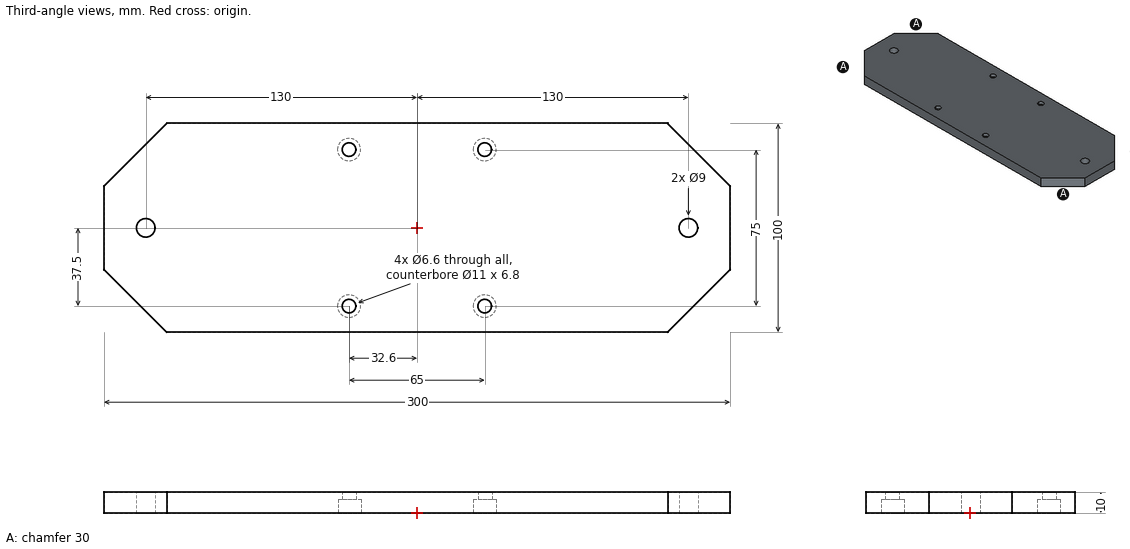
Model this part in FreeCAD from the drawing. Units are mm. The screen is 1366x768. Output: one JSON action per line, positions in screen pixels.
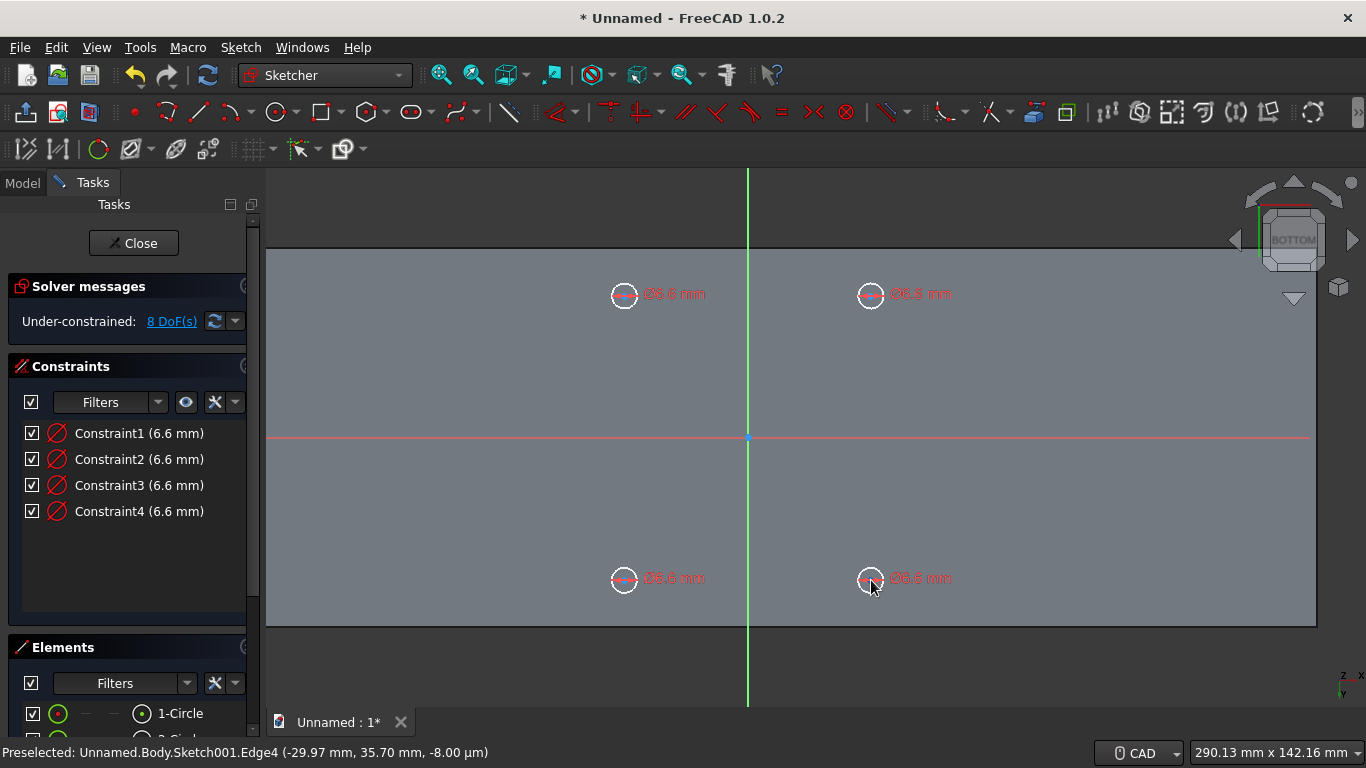
{"action": "left_click", "coordinate": [625, 296]}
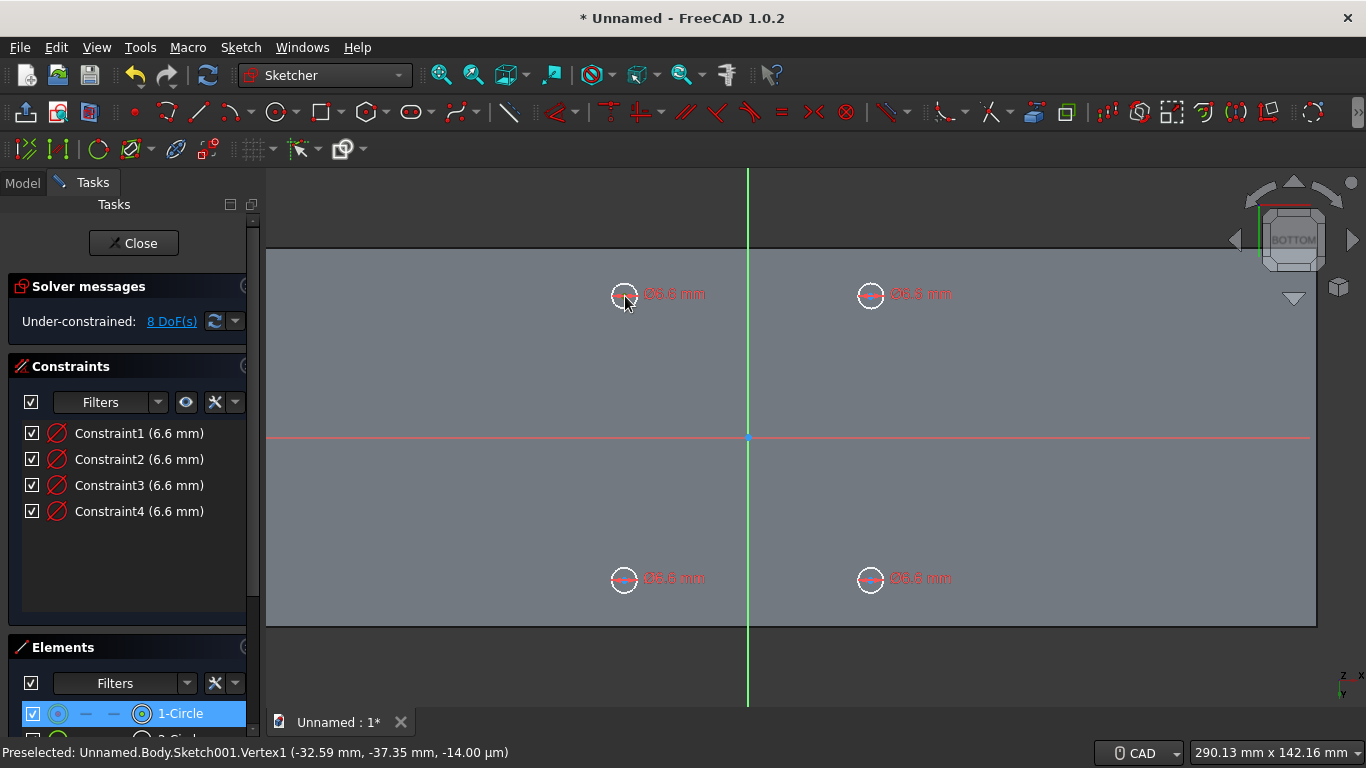
{"action": "left_click", "coordinate": [871, 296]}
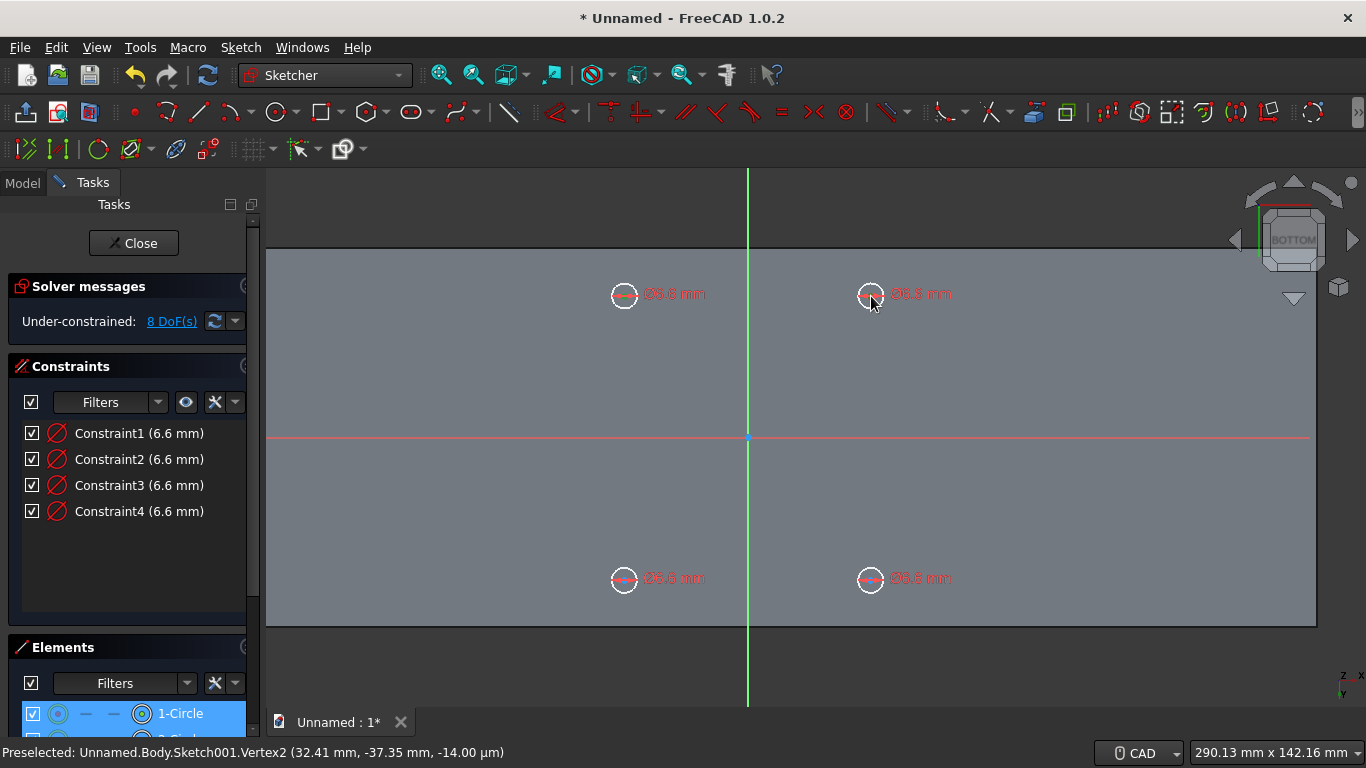
{"action": "key", "text": "h"}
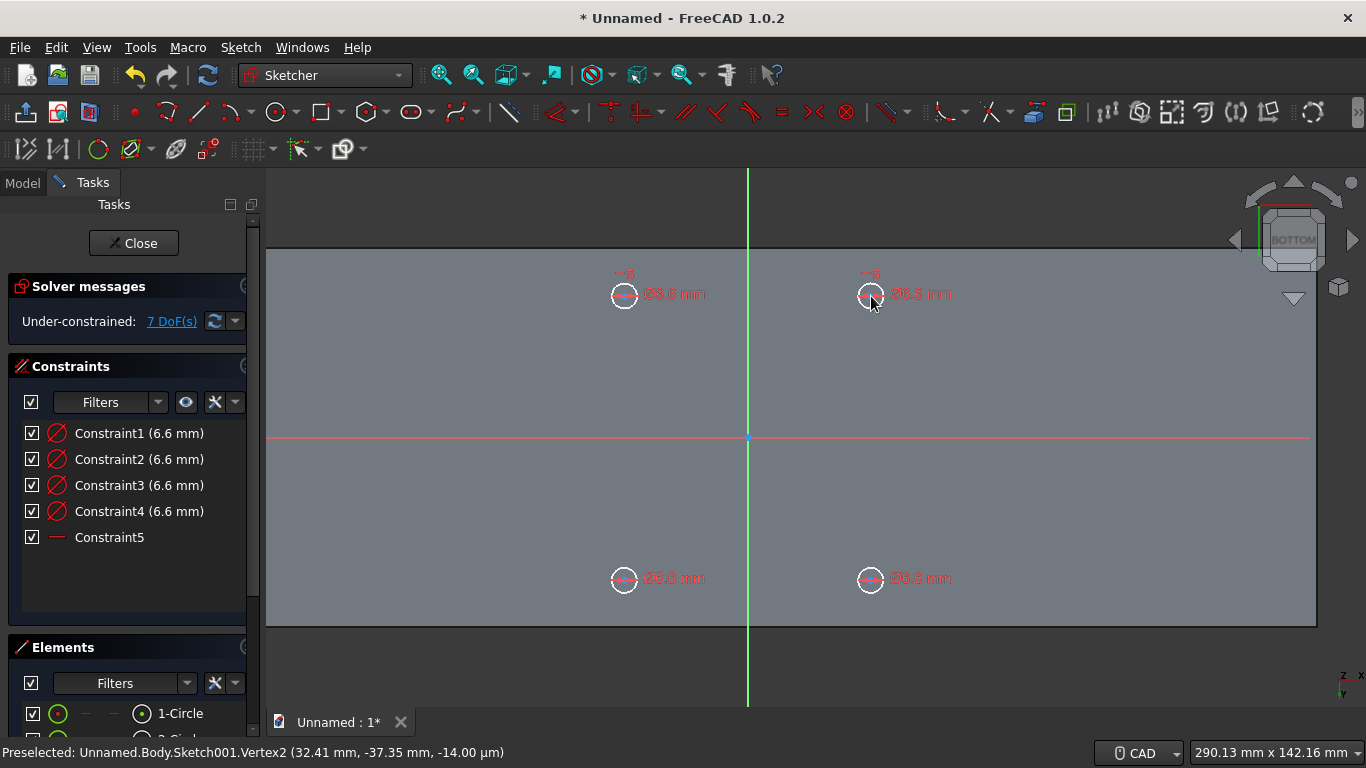
{"action": "left_click", "coordinate": [871, 296]}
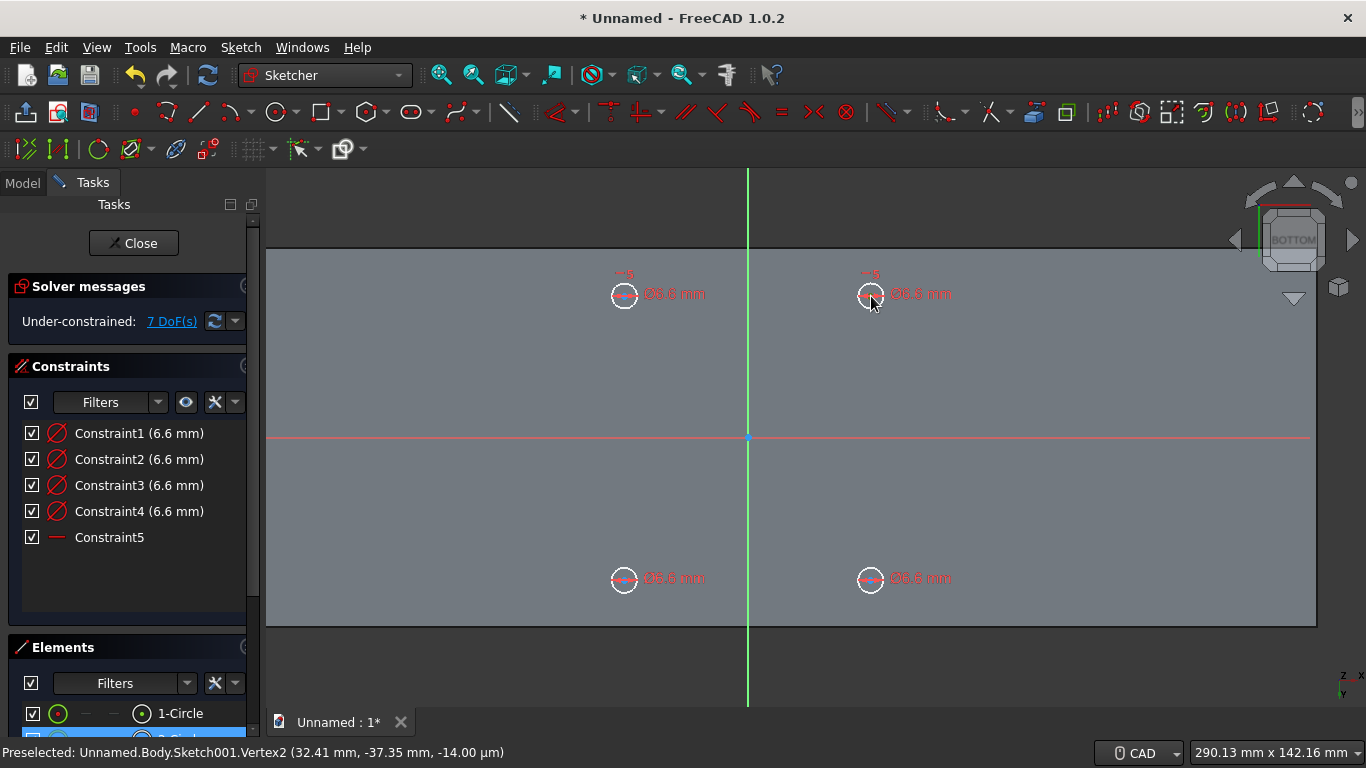
{"action": "left_click", "coordinate": [871, 580]}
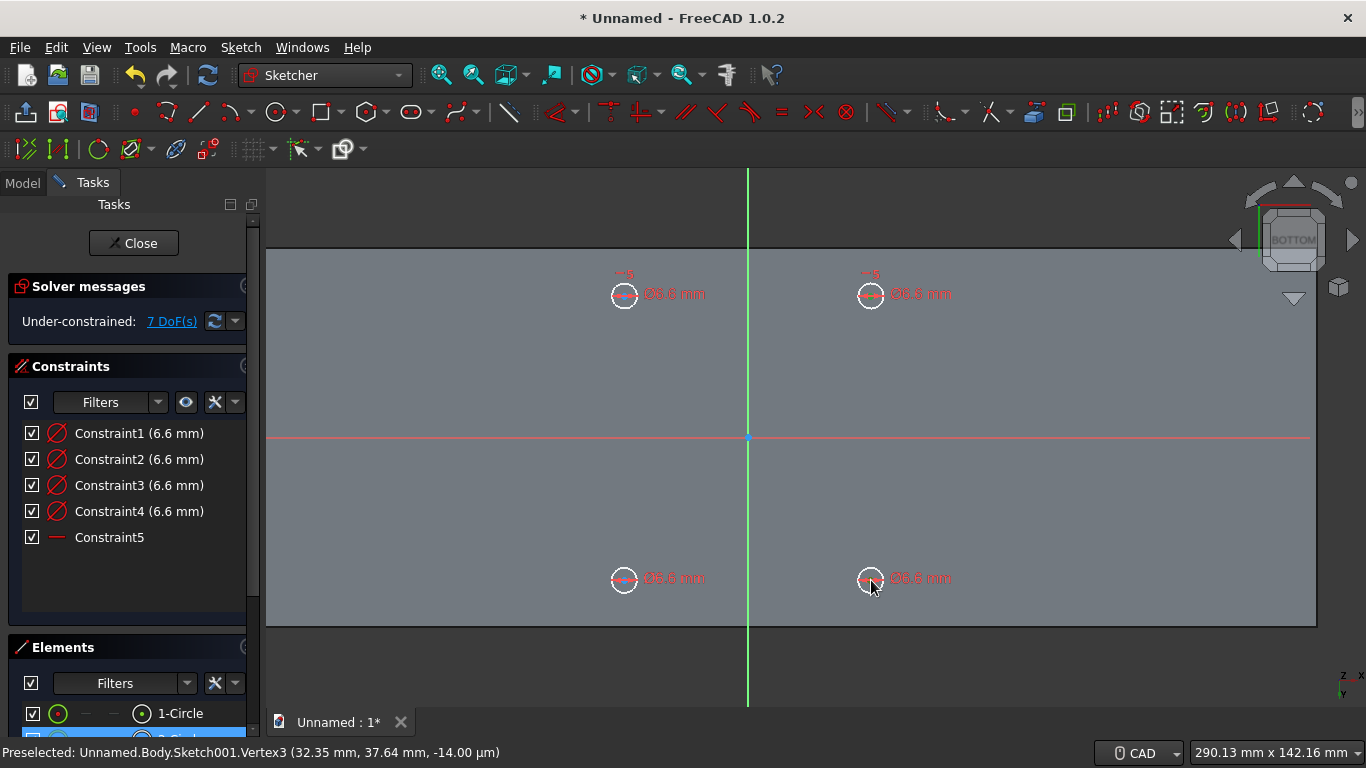
{"action": "key", "text": "v"}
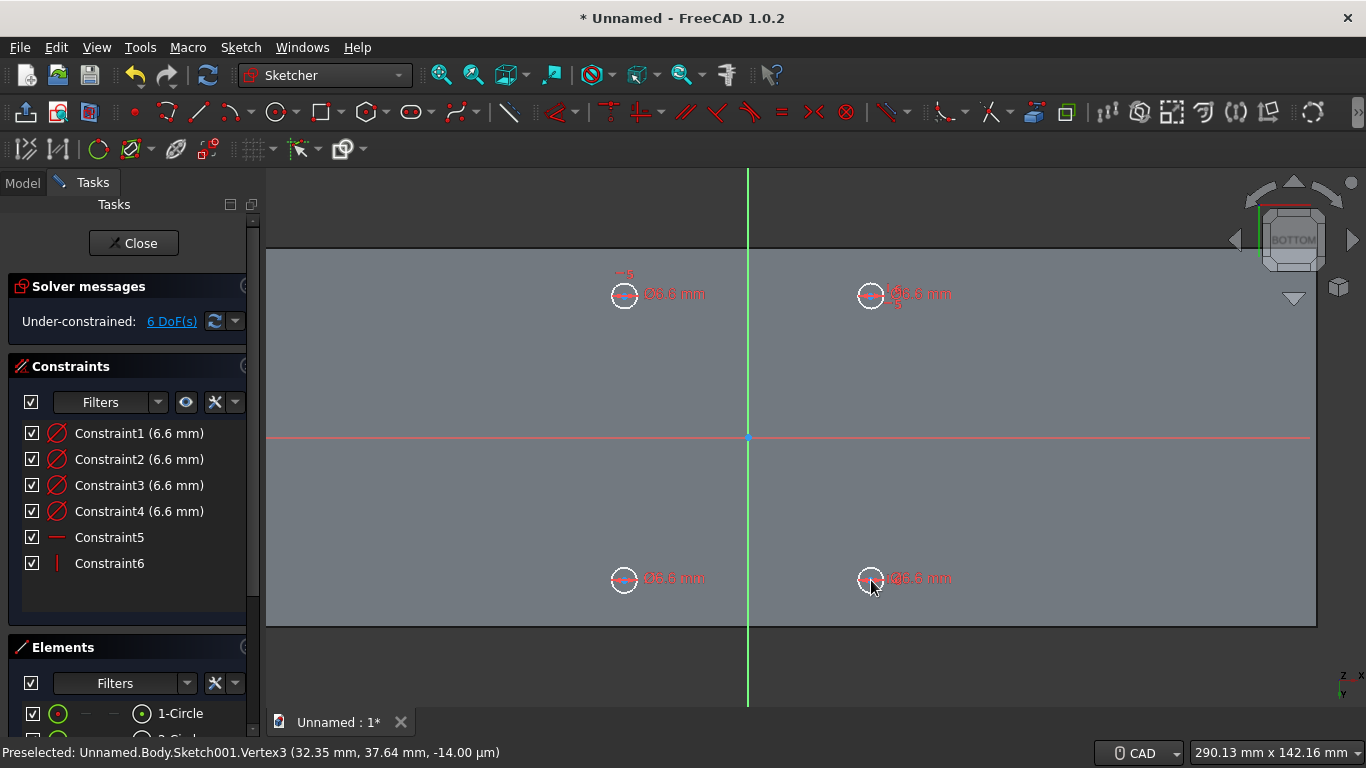
{"action": "left_click", "coordinate": [625, 296]}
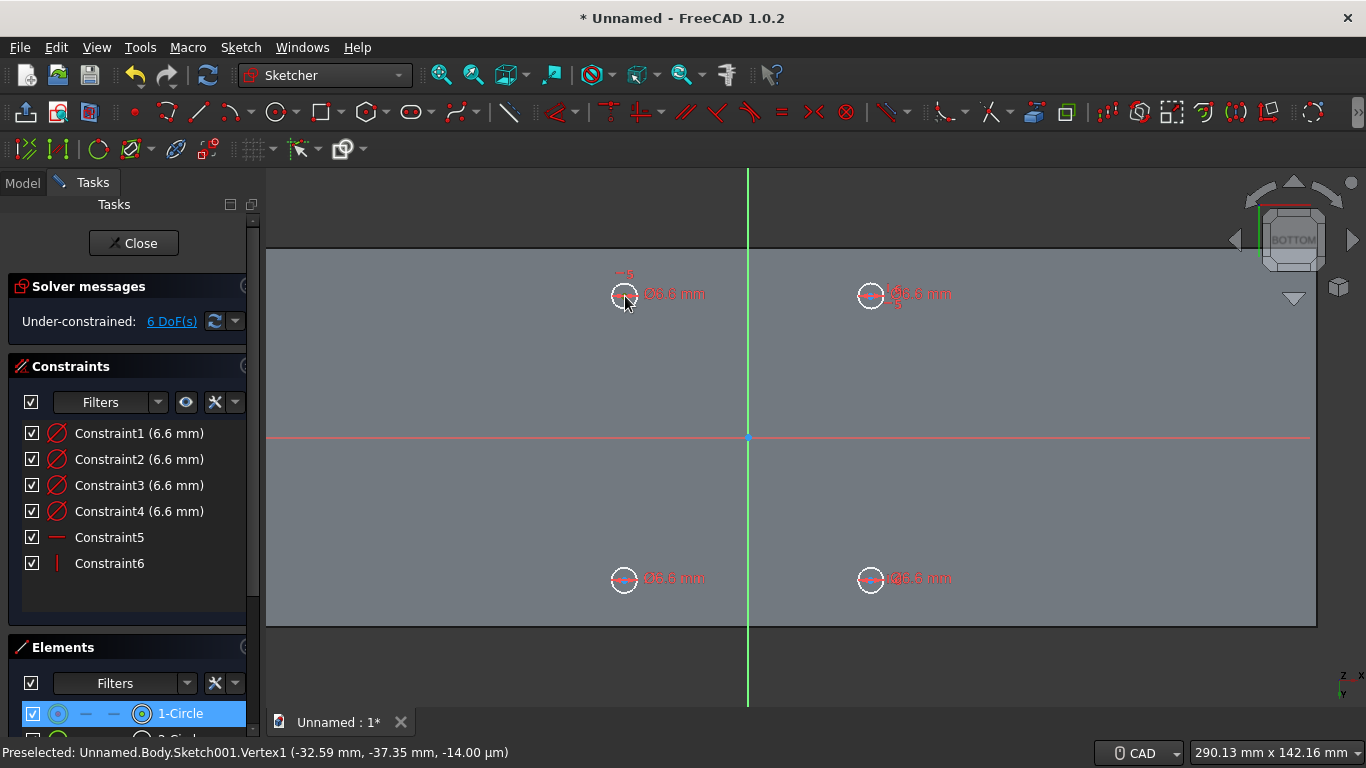
{"action": "left_click", "coordinate": [624, 580]}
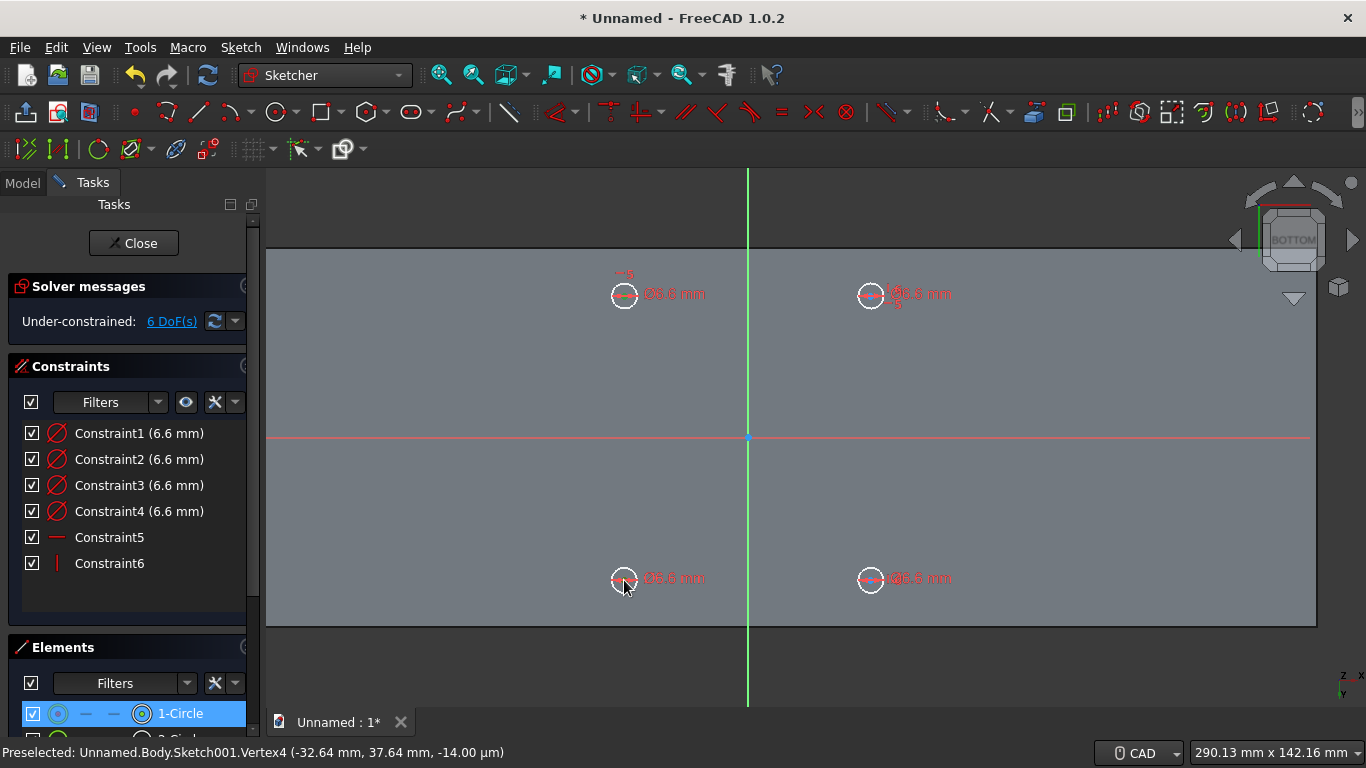
{"action": "key", "text": "v"}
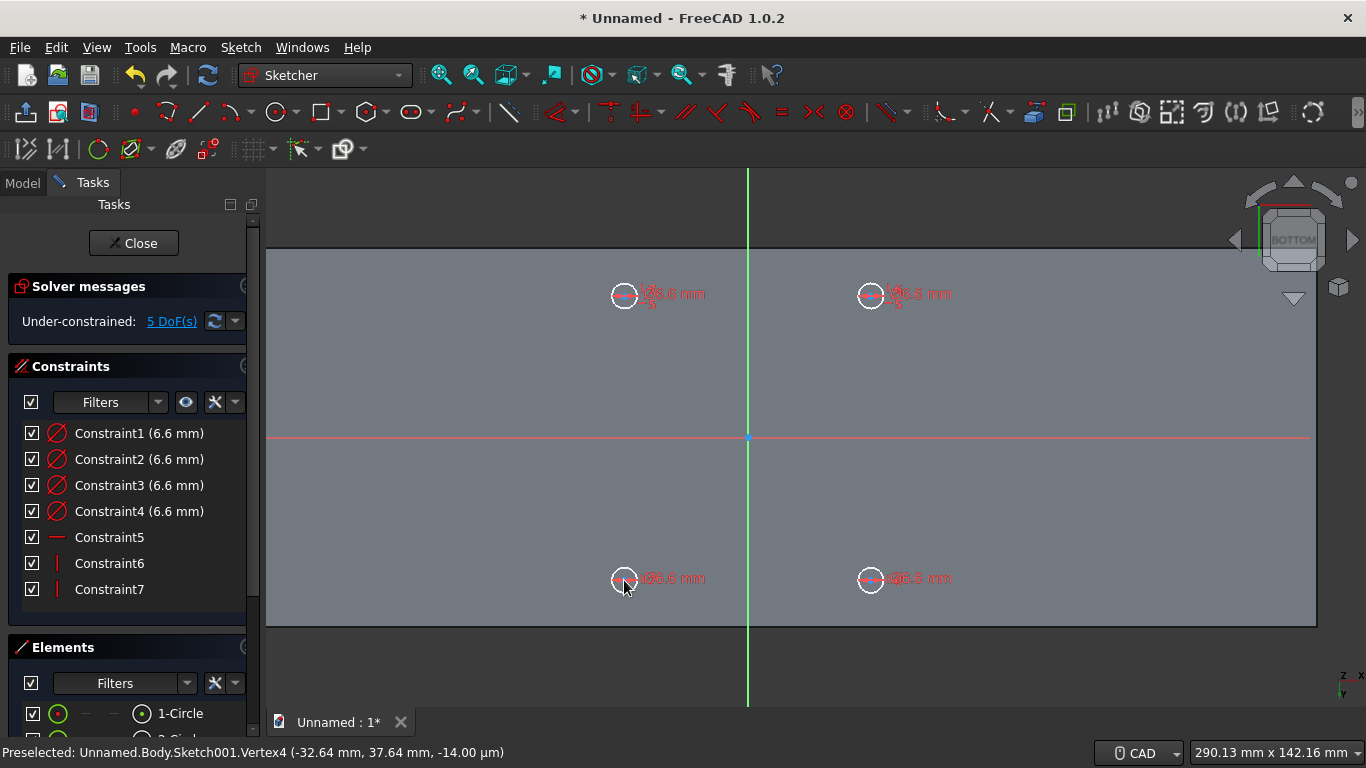
{"action": "left_click", "coordinate": [871, 580]}